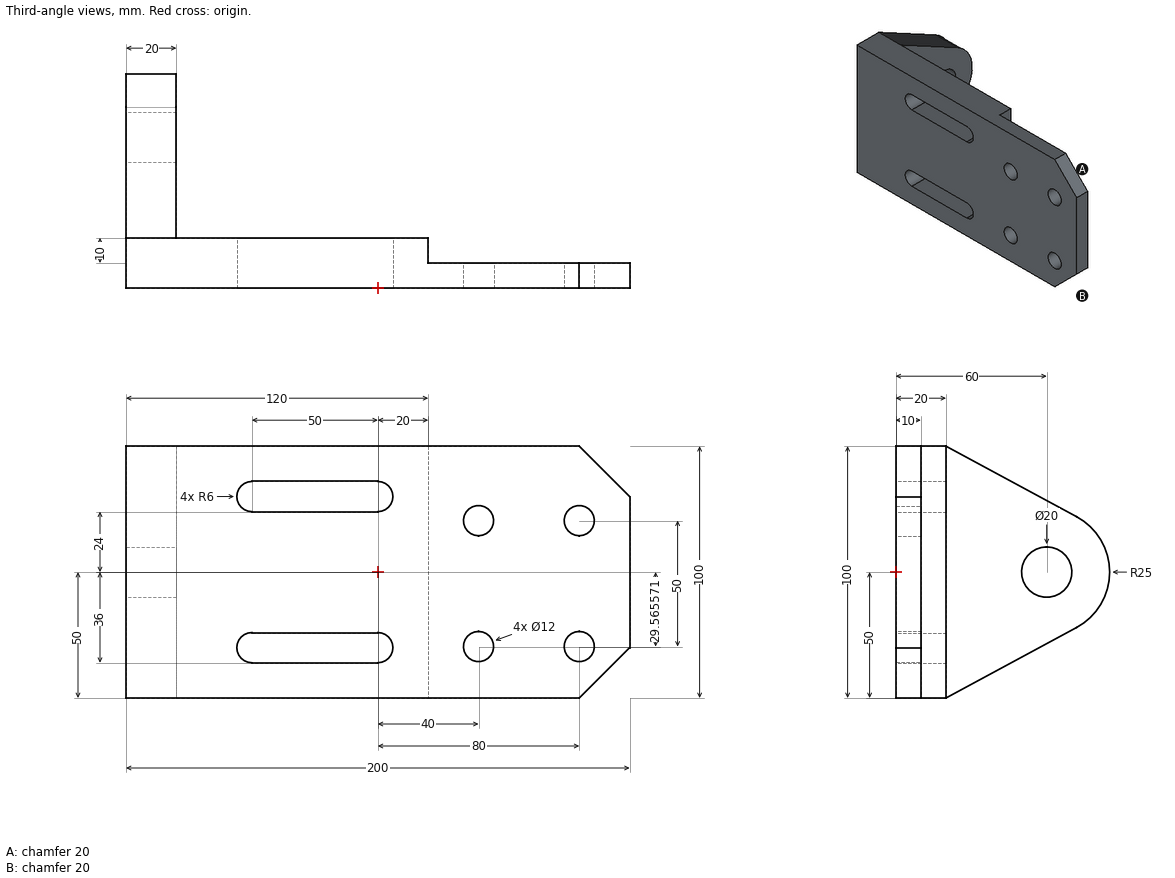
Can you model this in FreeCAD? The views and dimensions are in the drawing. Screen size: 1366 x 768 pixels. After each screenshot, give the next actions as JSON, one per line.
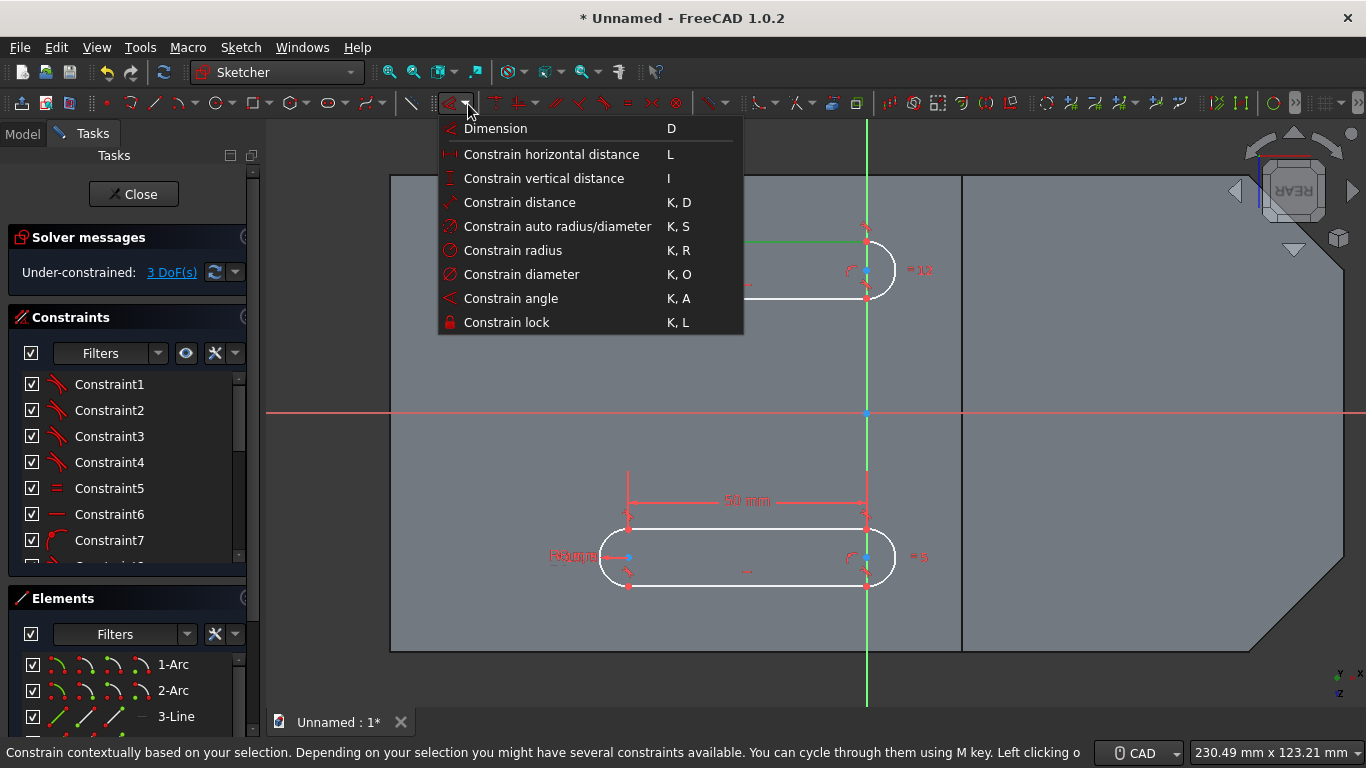
{"action": "left_click", "coordinate": [591, 154]}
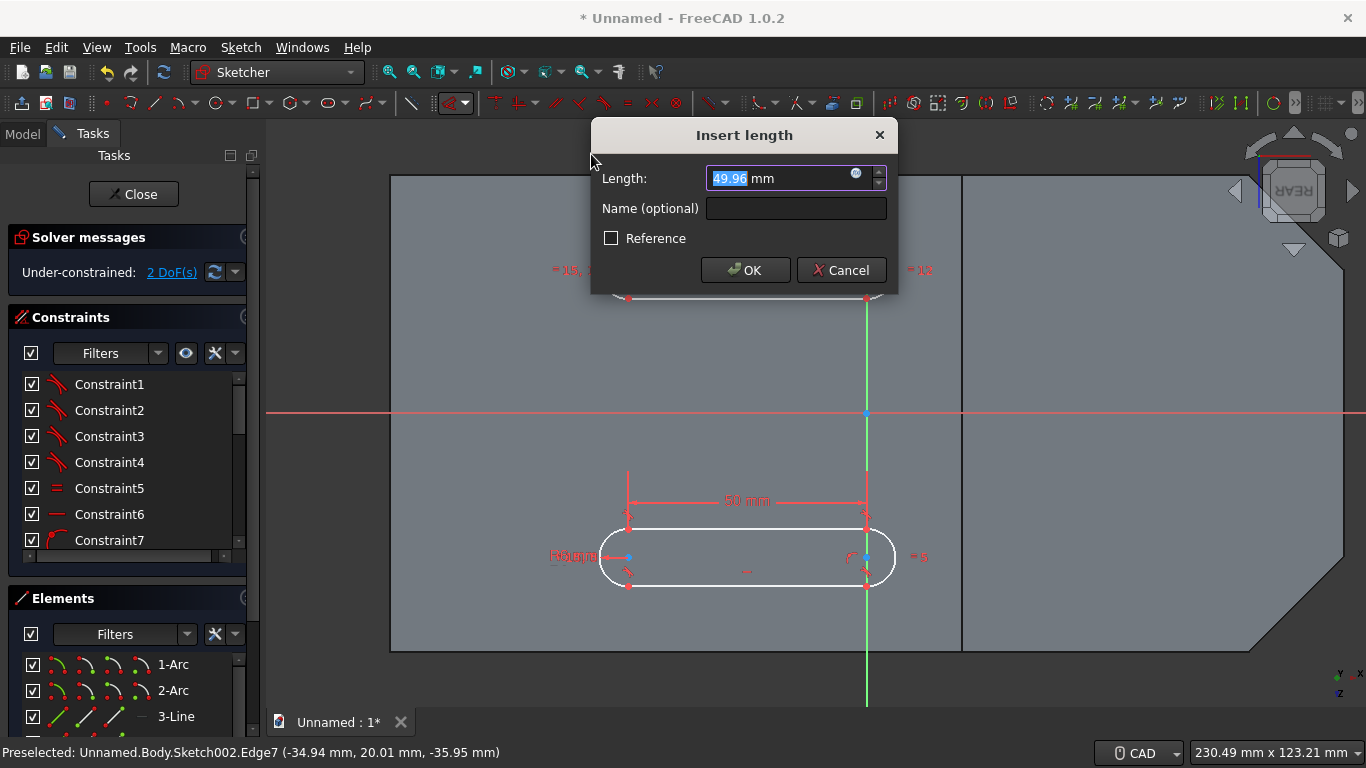
{"action": "type", "text": "50"}
{"action": "key", "text": "Return"}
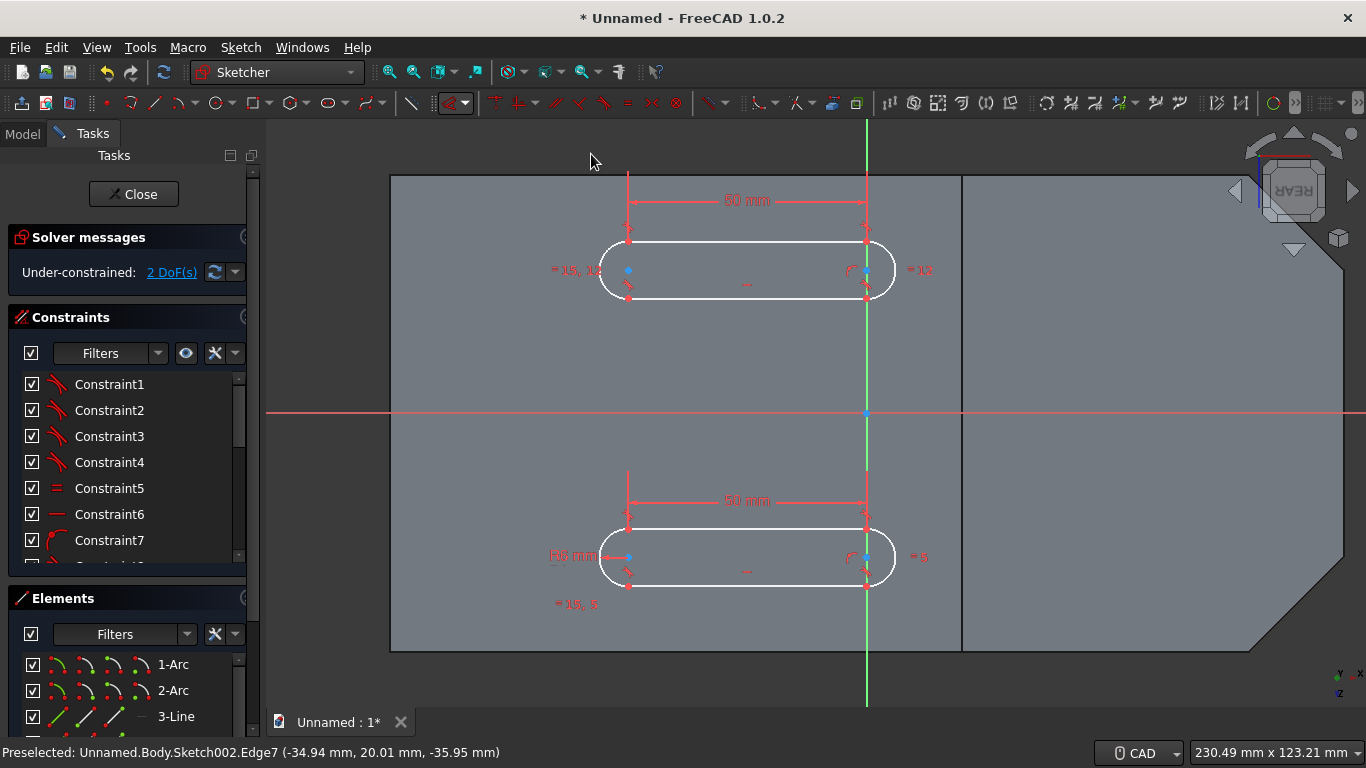
{"action": "left_click", "coordinate": [628, 529]}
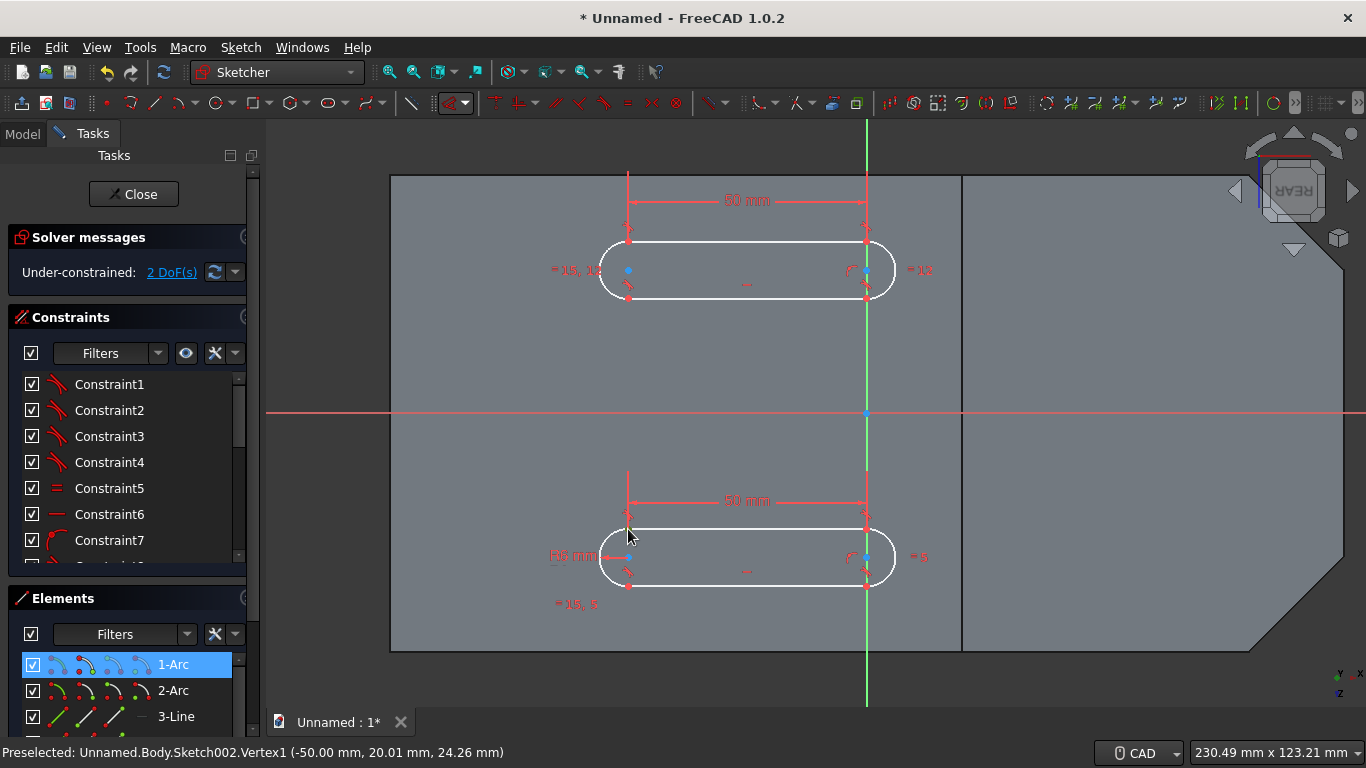
{"action": "left_click", "coordinate": [468, 104]}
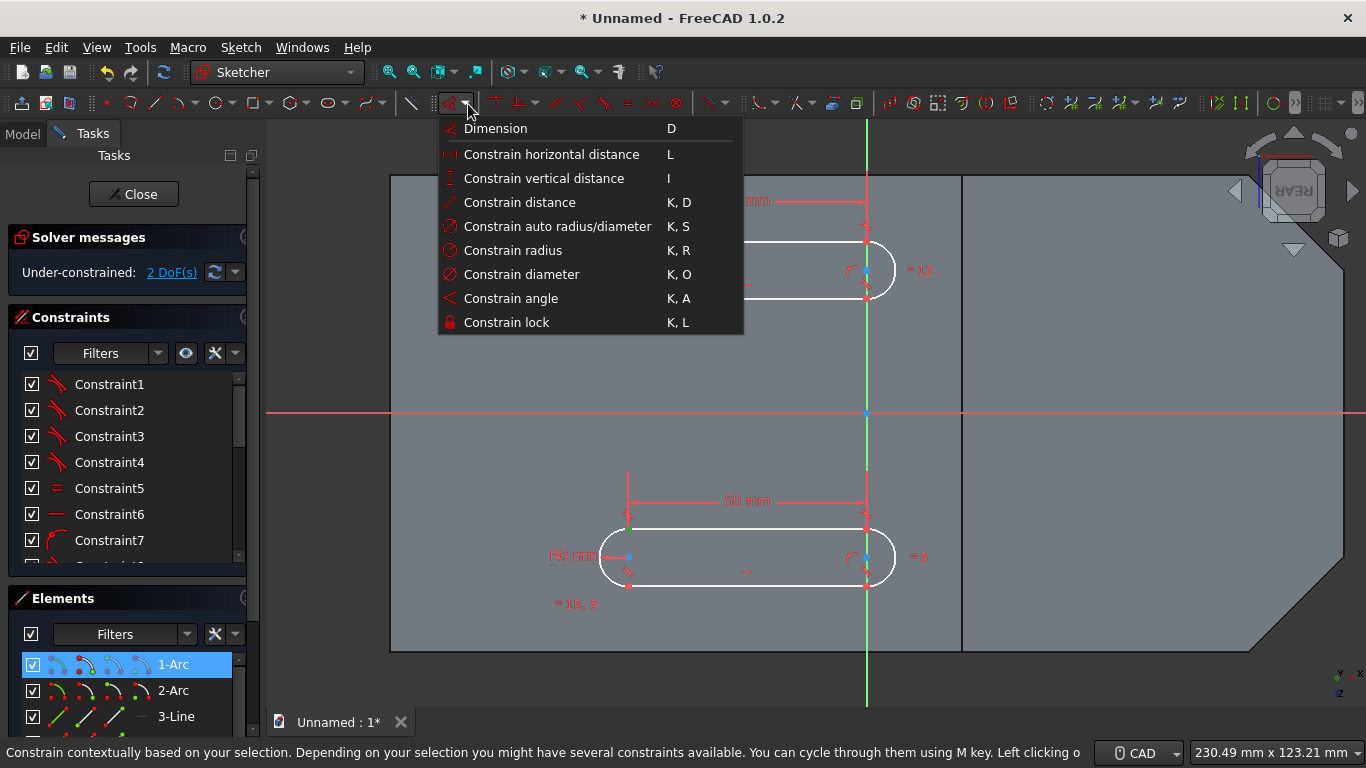
{"action": "left_click", "coordinate": [591, 178]}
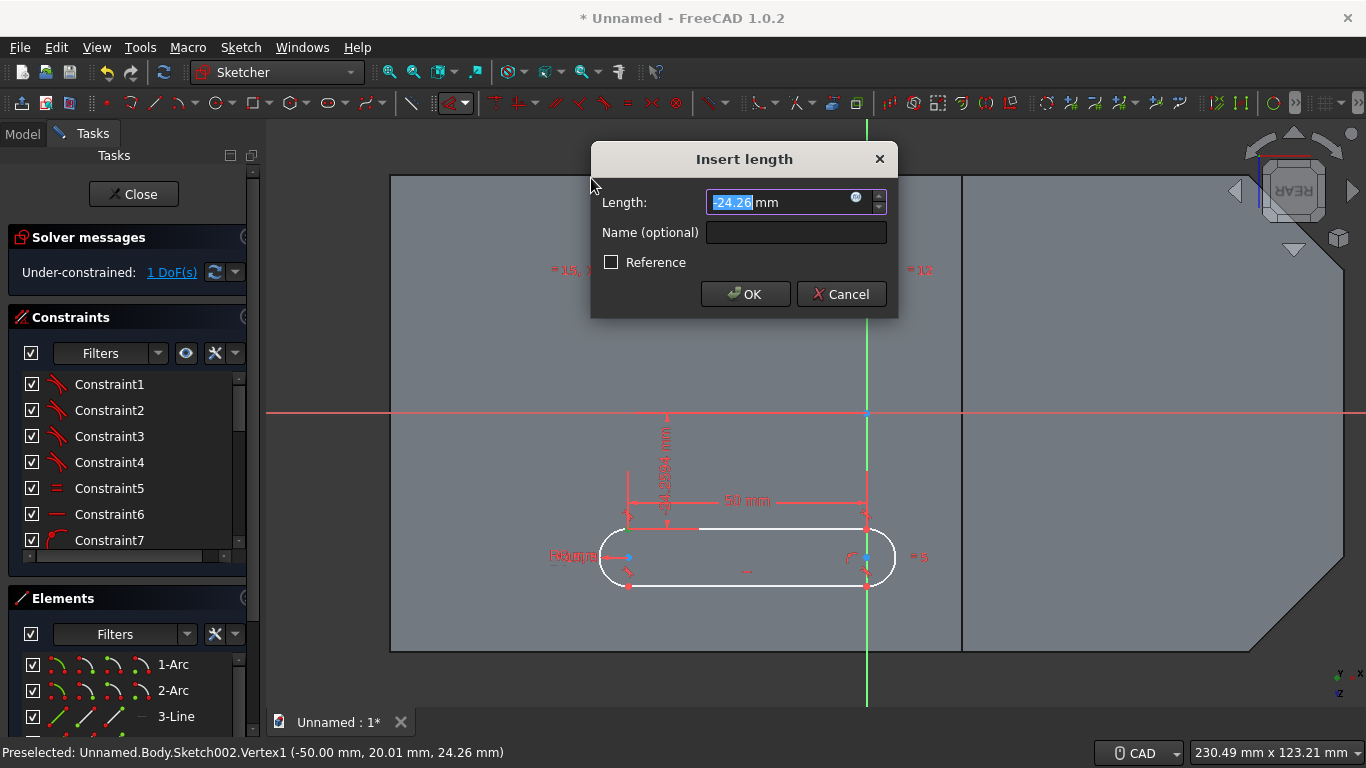
{"action": "type", "text": "-24"}
{"action": "key", "text": "Return"}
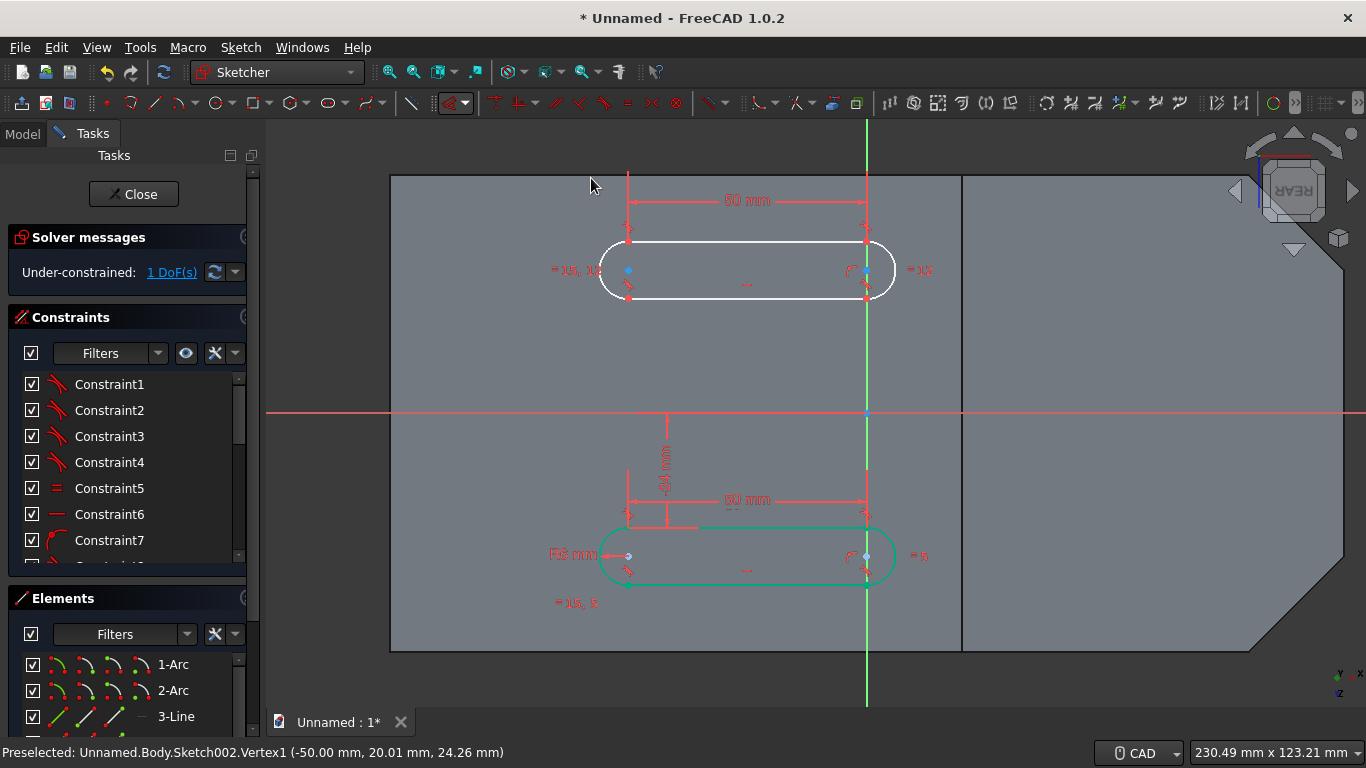
{"action": "left_click", "coordinate": [628, 242]}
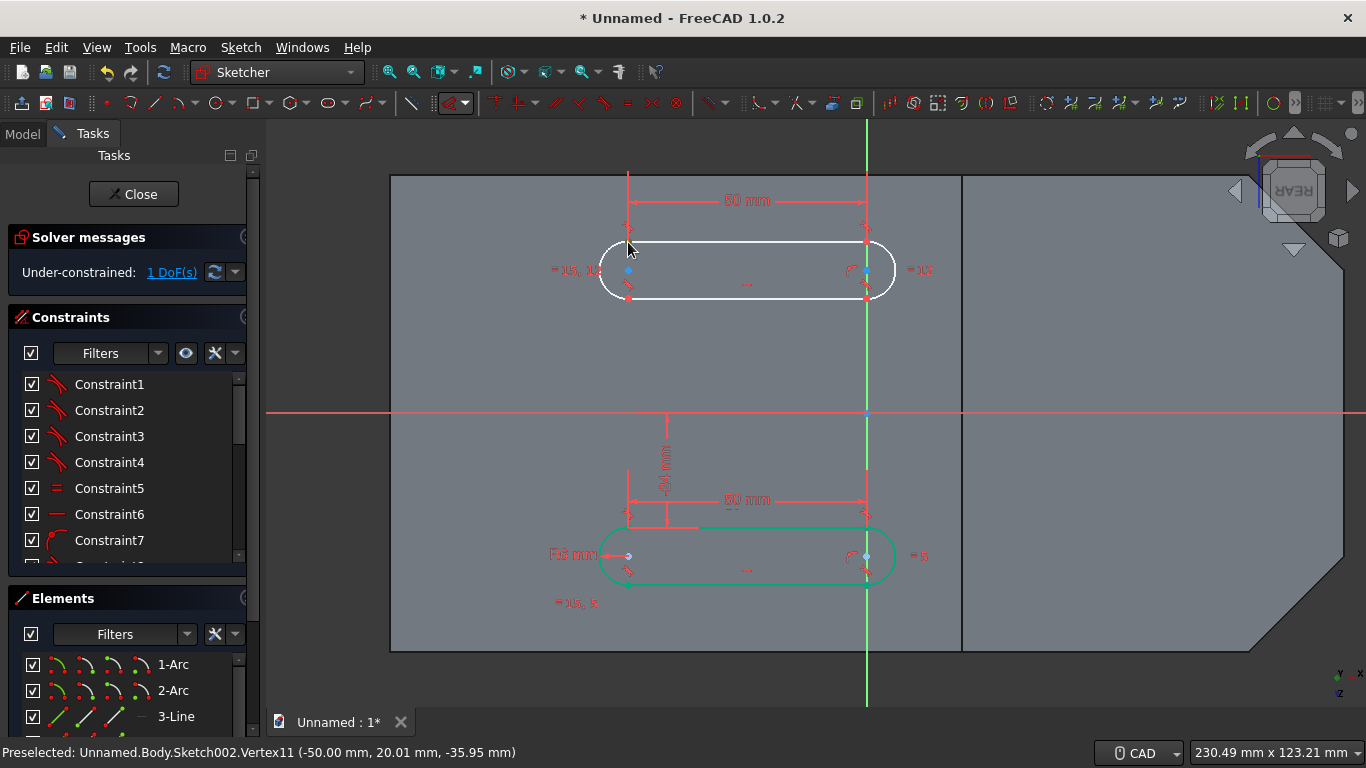
{"action": "left_click", "coordinate": [468, 104]}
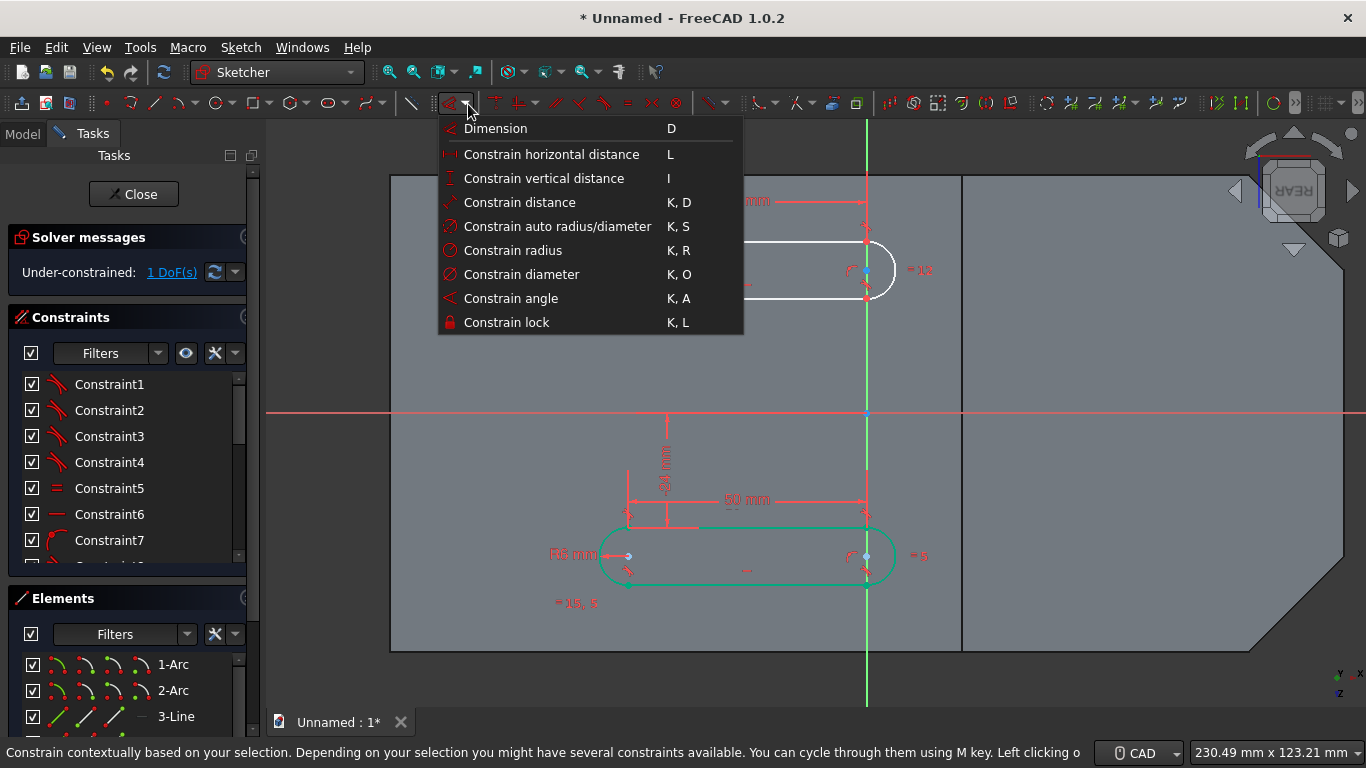
{"action": "left_click", "coordinate": [591, 178]}